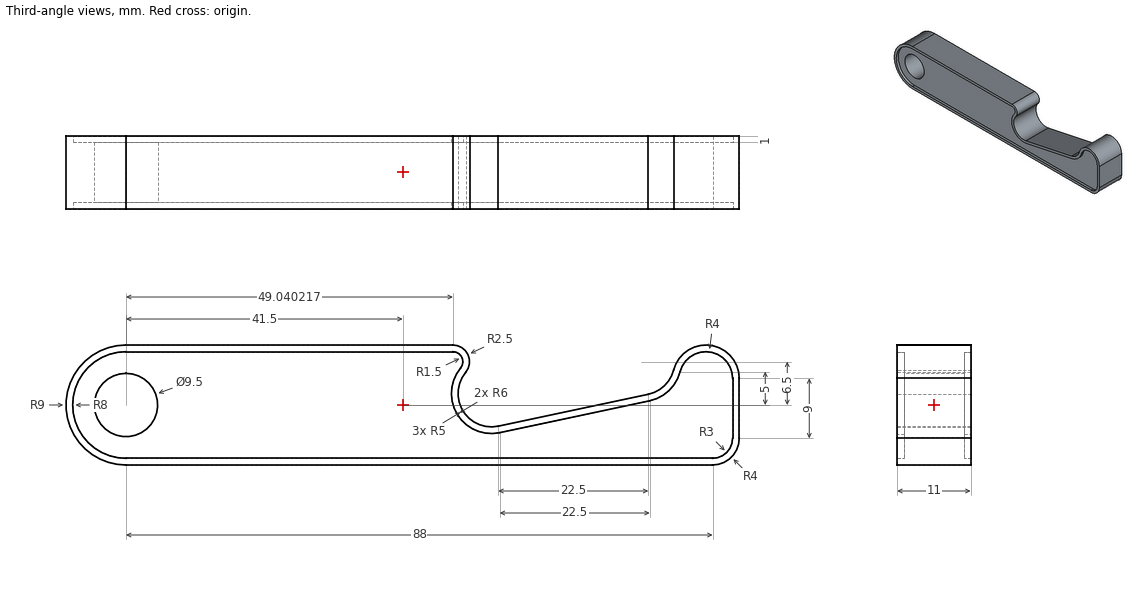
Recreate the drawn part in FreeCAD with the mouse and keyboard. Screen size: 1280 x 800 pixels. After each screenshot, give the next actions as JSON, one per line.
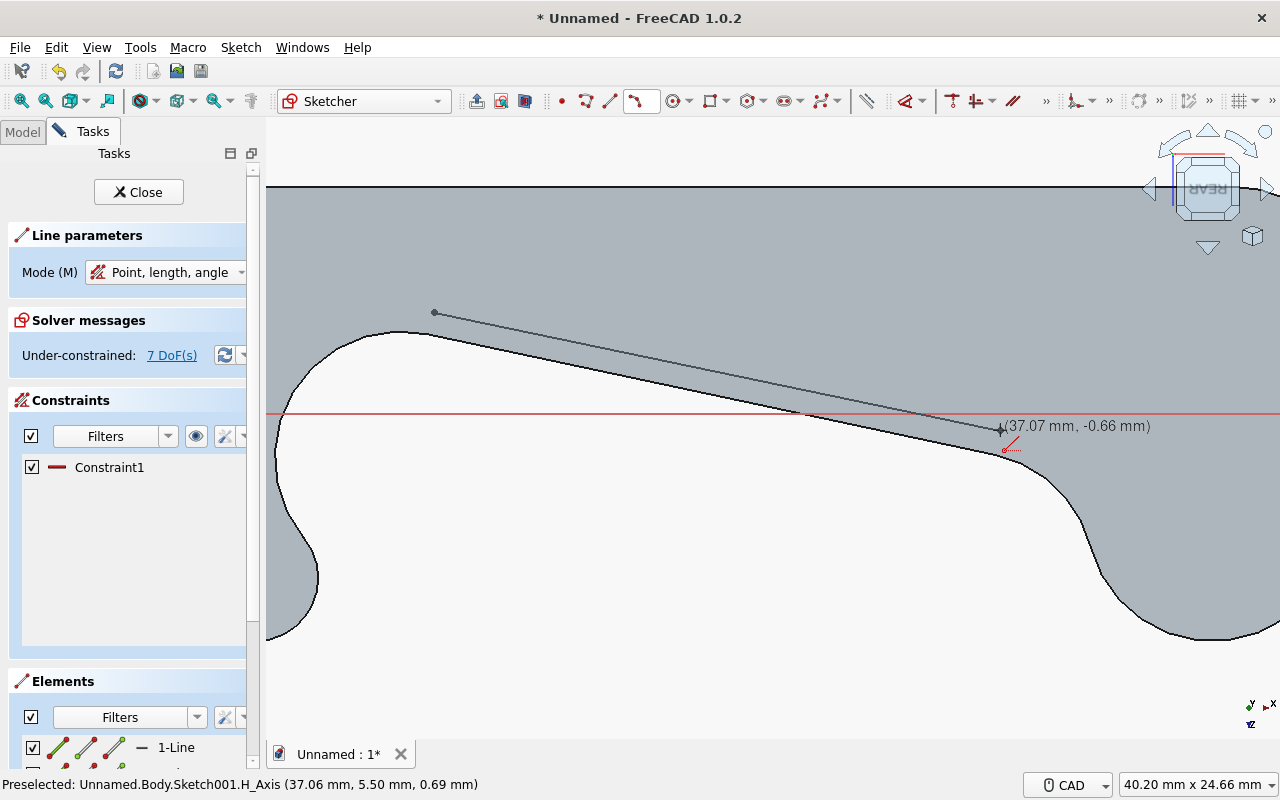
{"action": "scroll", "coordinate": [914, 433], "scroll_direction": "down", "scroll_amount": 7}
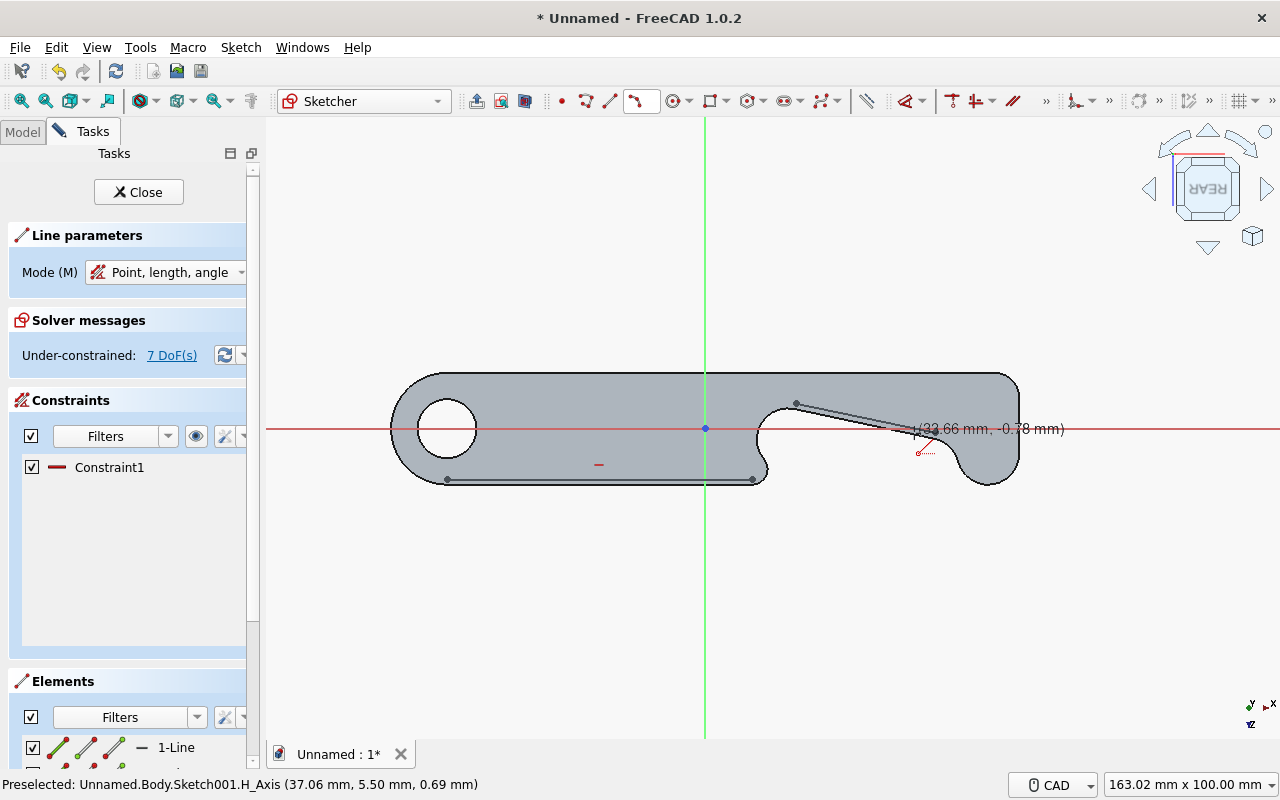
{"action": "left_click", "coordinate": [1013, 454]}
{"action": "left_click", "coordinate": [1013, 398]}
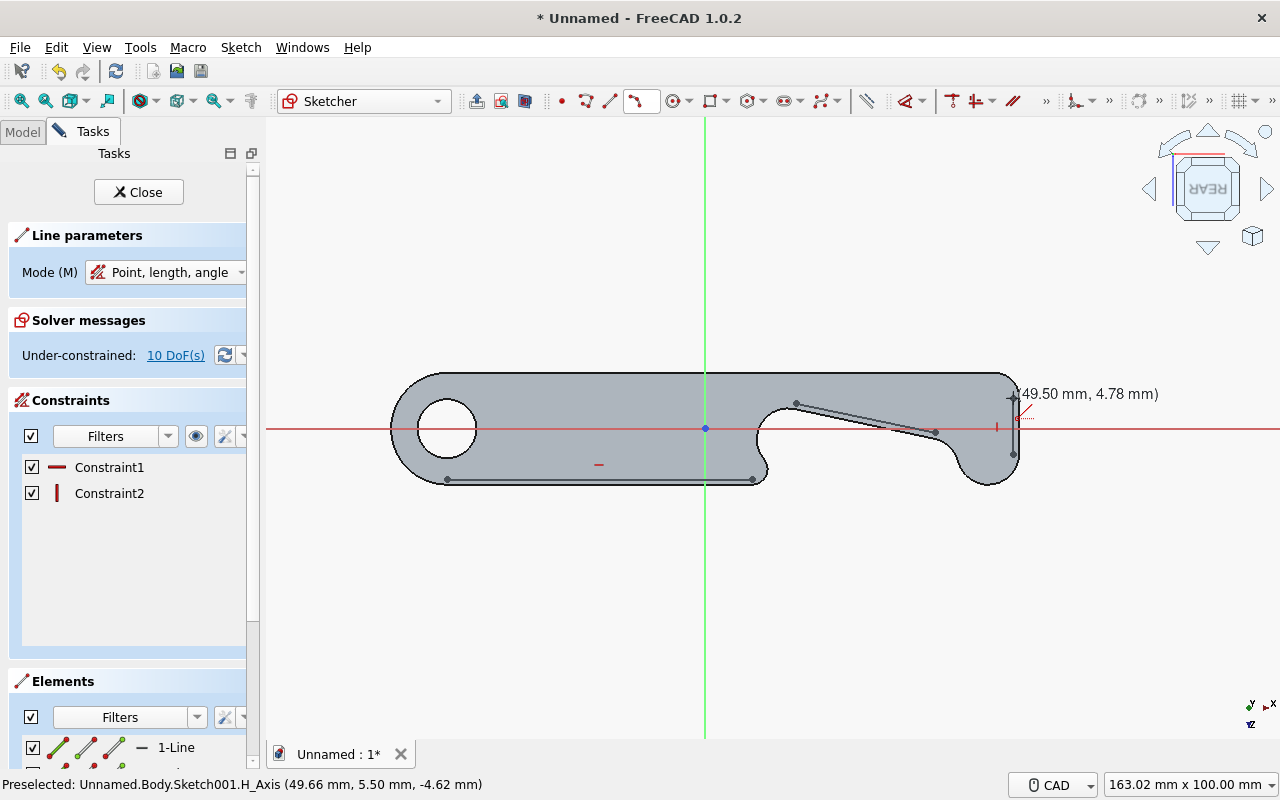
{"action": "left_click", "coordinate": [994, 379]}
{"action": "left_click", "coordinate": [447, 379]}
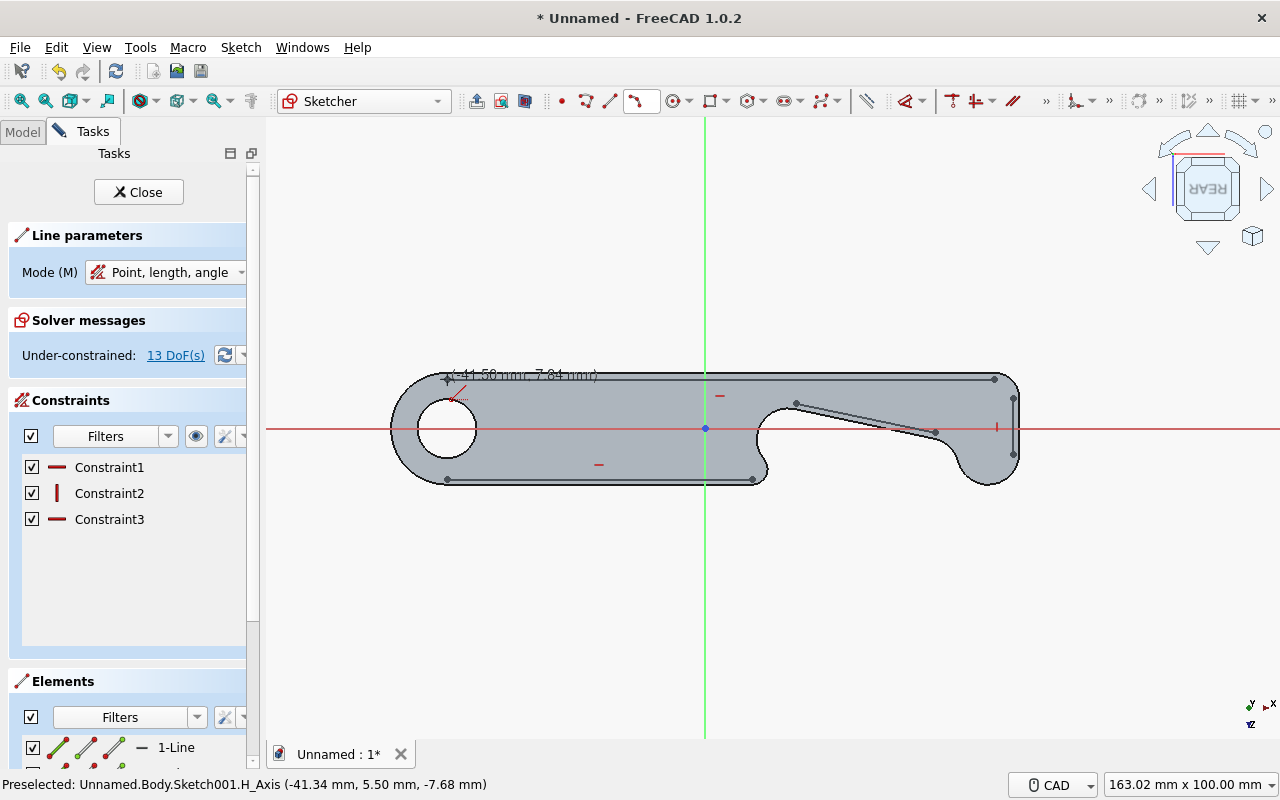
{"action": "left_click", "coordinate": [636, 102]}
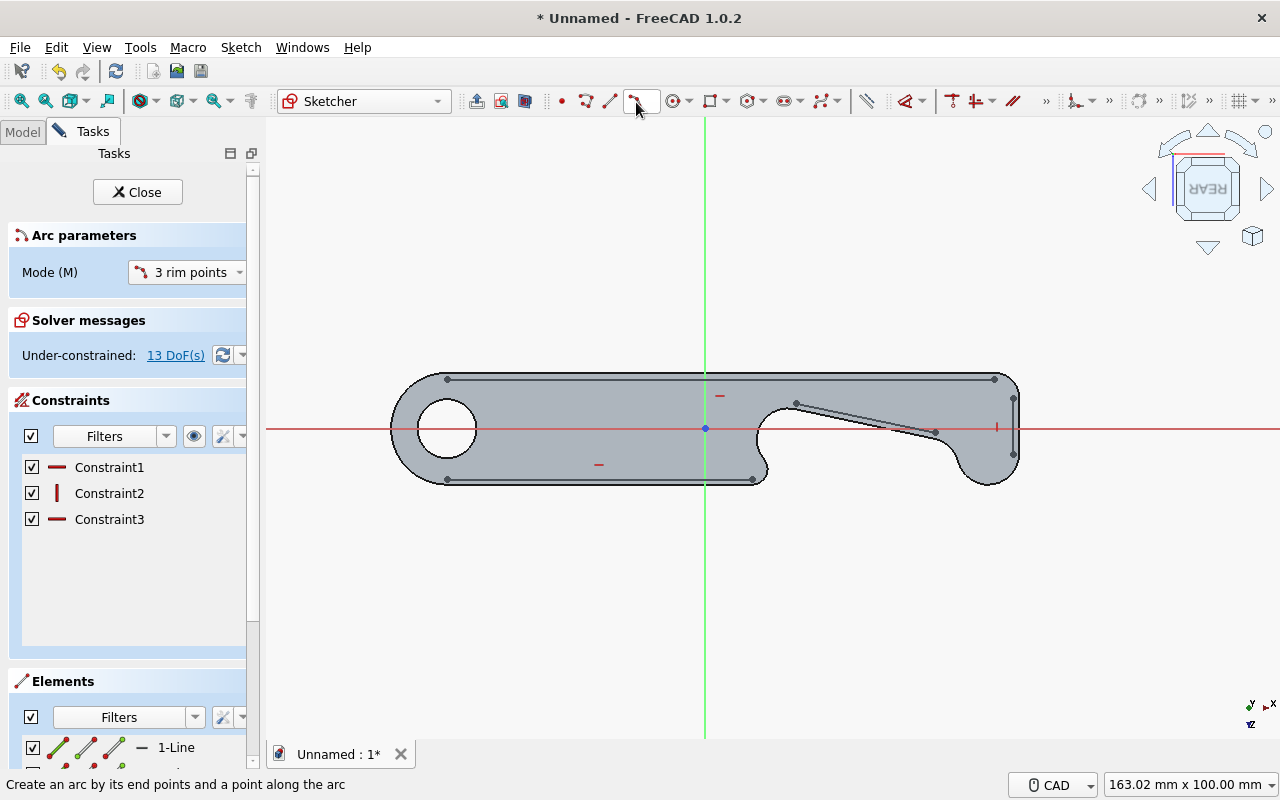
{"action": "left_click", "coordinate": [752, 480]}
{"action": "left_click", "coordinate": [759, 463]}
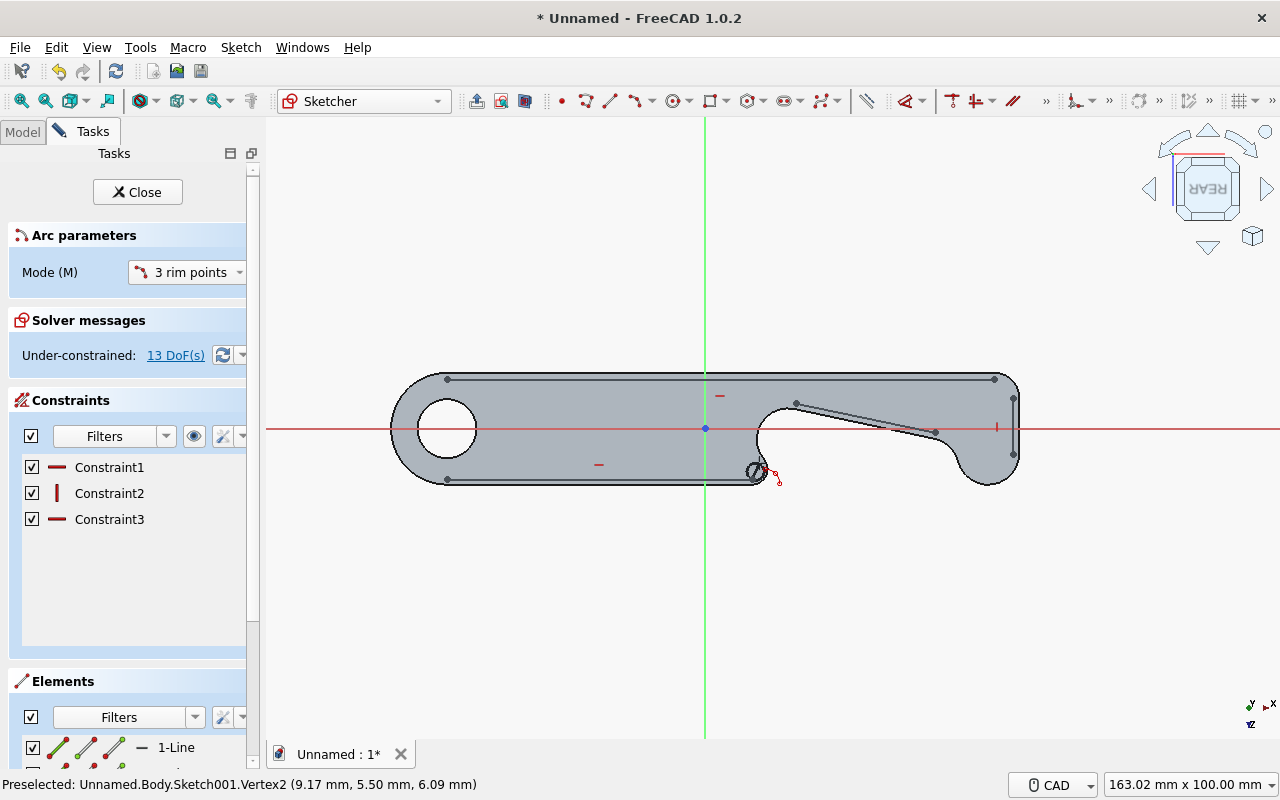
{"action": "scroll", "coordinate": [760, 473], "scroll_direction": "up", "scroll_amount": 6}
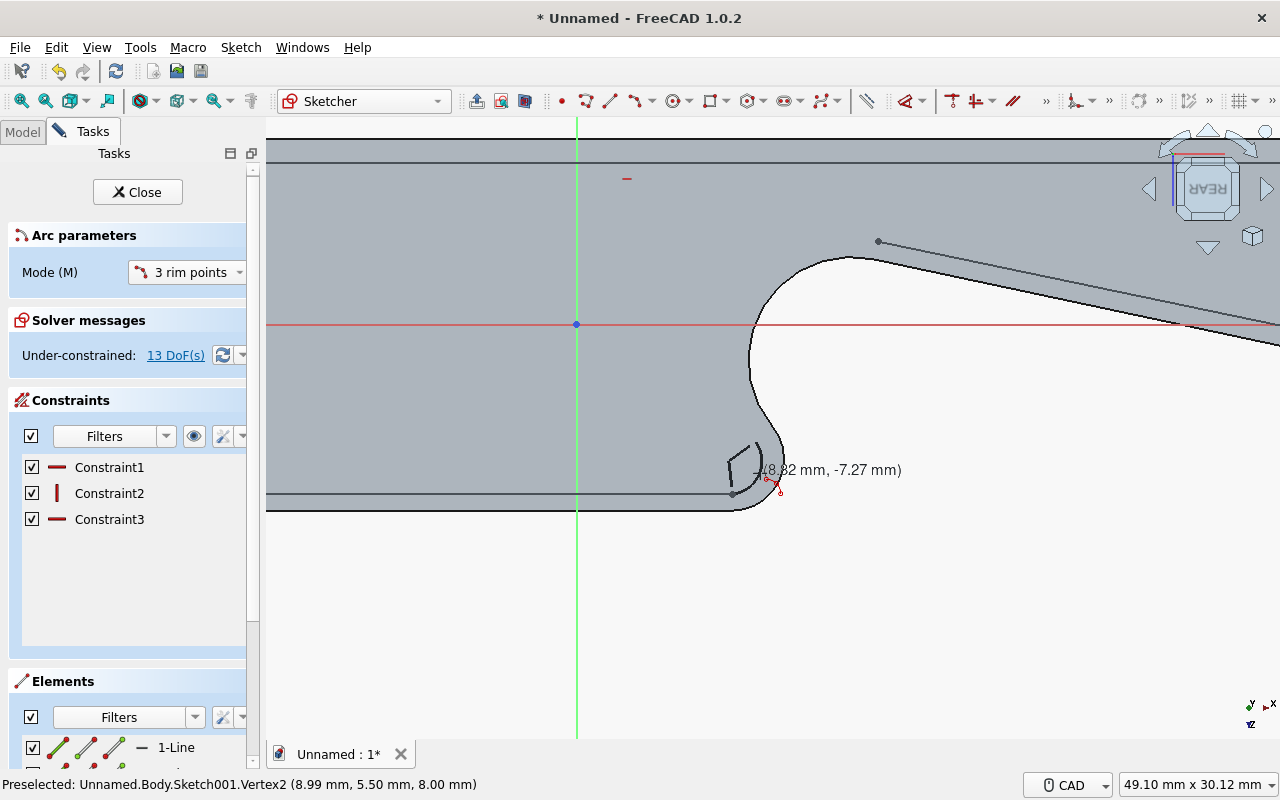
{"action": "left_click", "coordinate": [760, 472]}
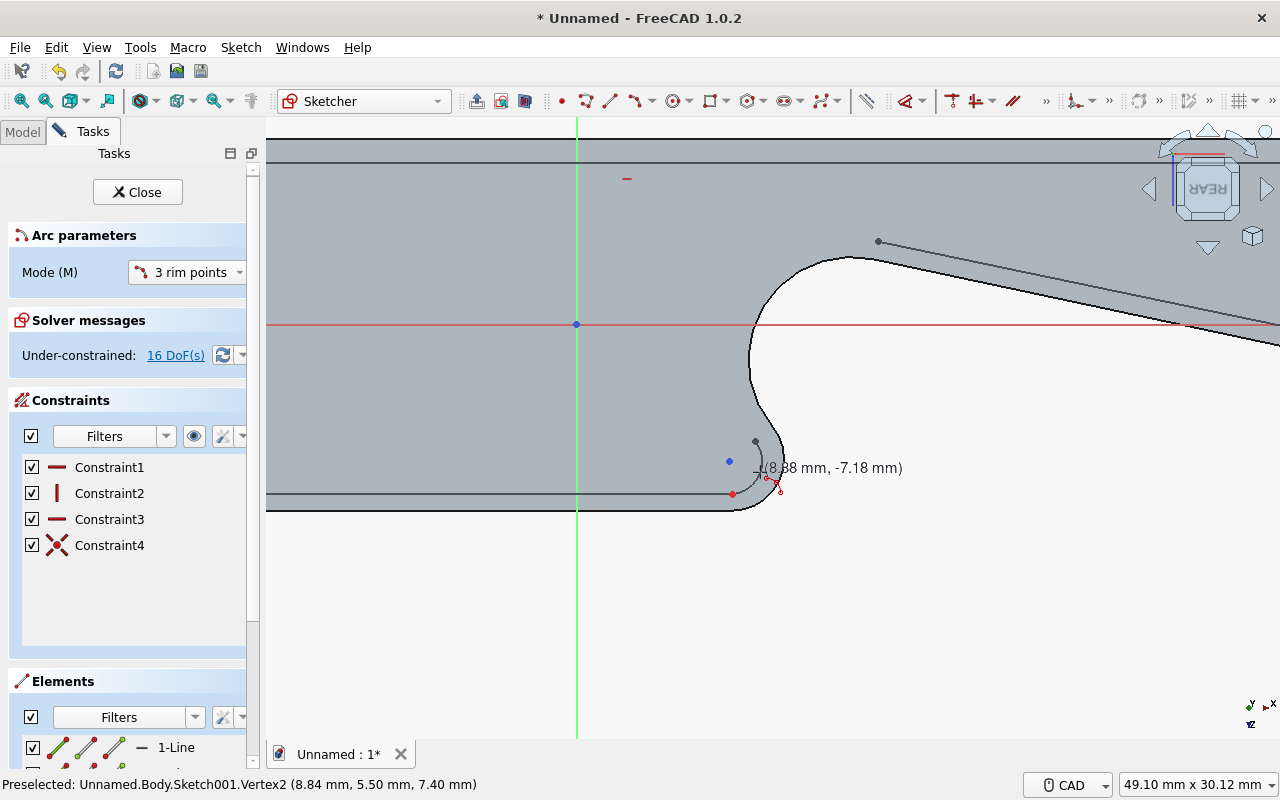
{"action": "left_click", "coordinate": [756, 442]}
{"action": "left_click", "coordinate": [879, 242]}
{"action": "left_click", "coordinate": [765, 272]}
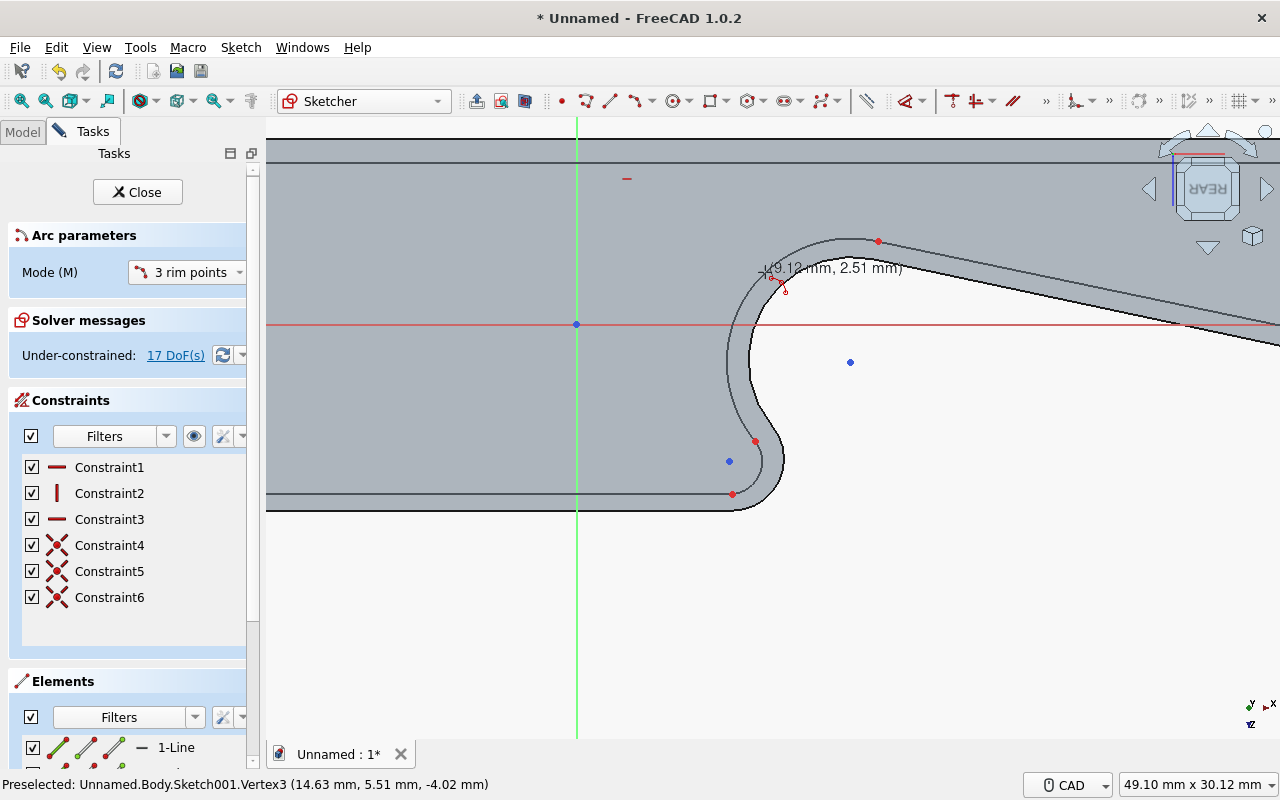
{"action": "scroll", "coordinate": [760, 472], "scroll_direction": "down", "scroll_amount": 6}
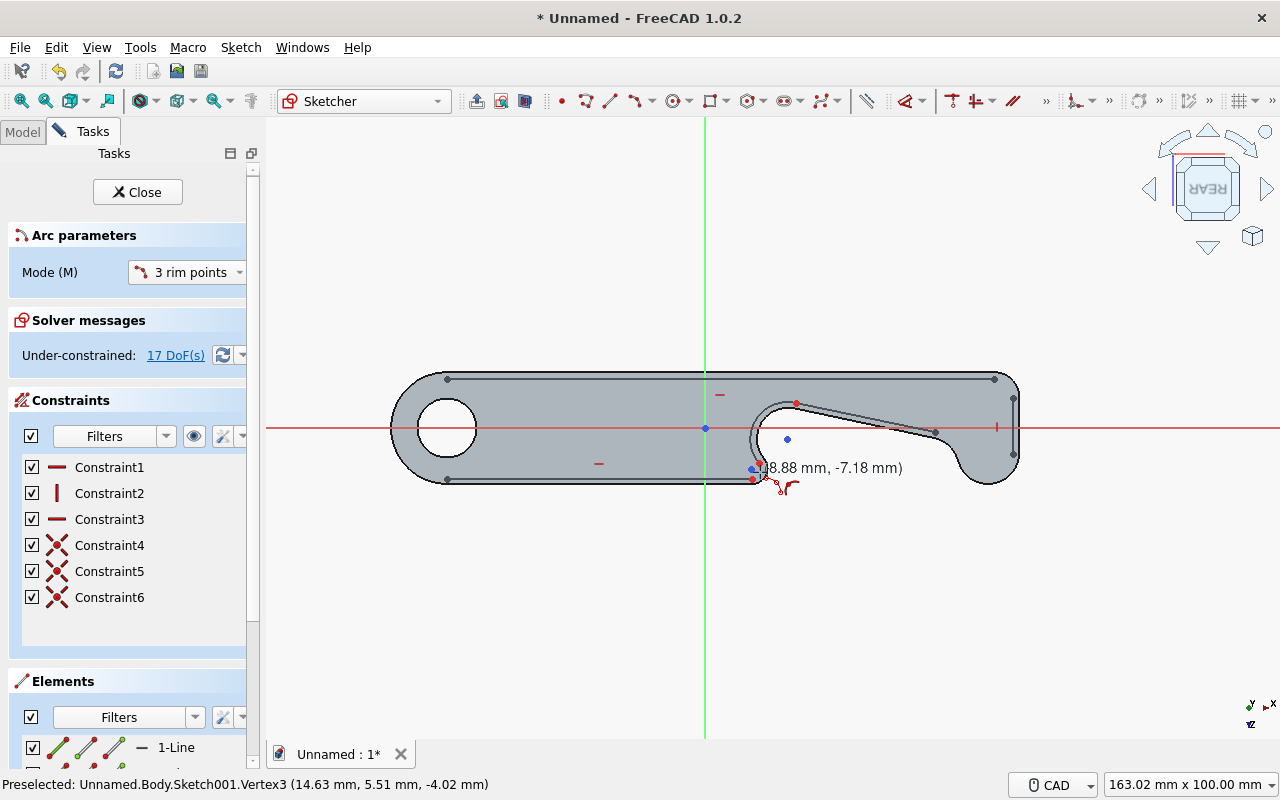
{"action": "scroll", "coordinate": [936, 432], "scroll_direction": "up", "scroll_amount": 7}